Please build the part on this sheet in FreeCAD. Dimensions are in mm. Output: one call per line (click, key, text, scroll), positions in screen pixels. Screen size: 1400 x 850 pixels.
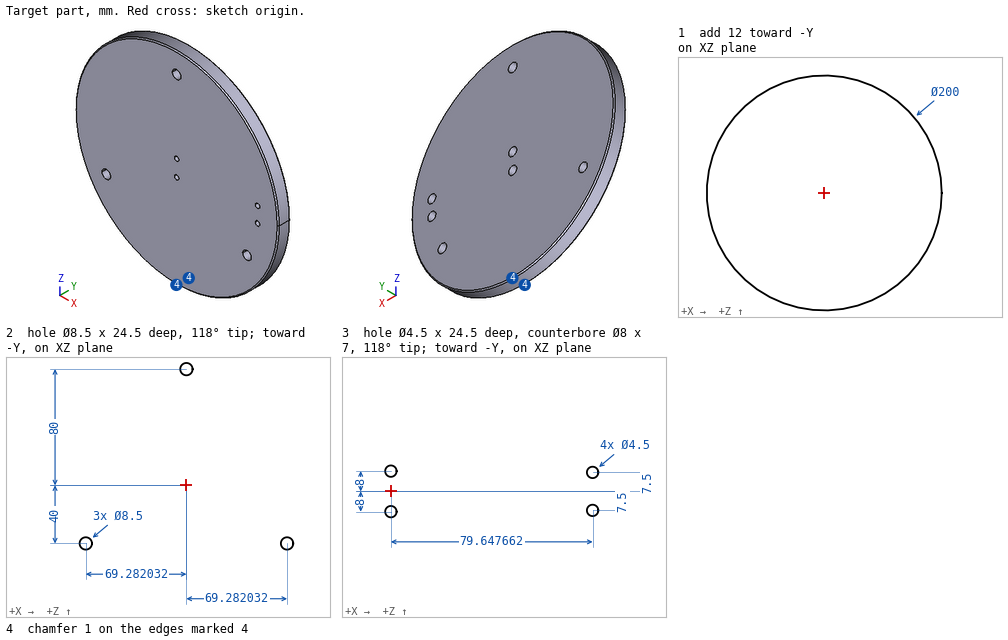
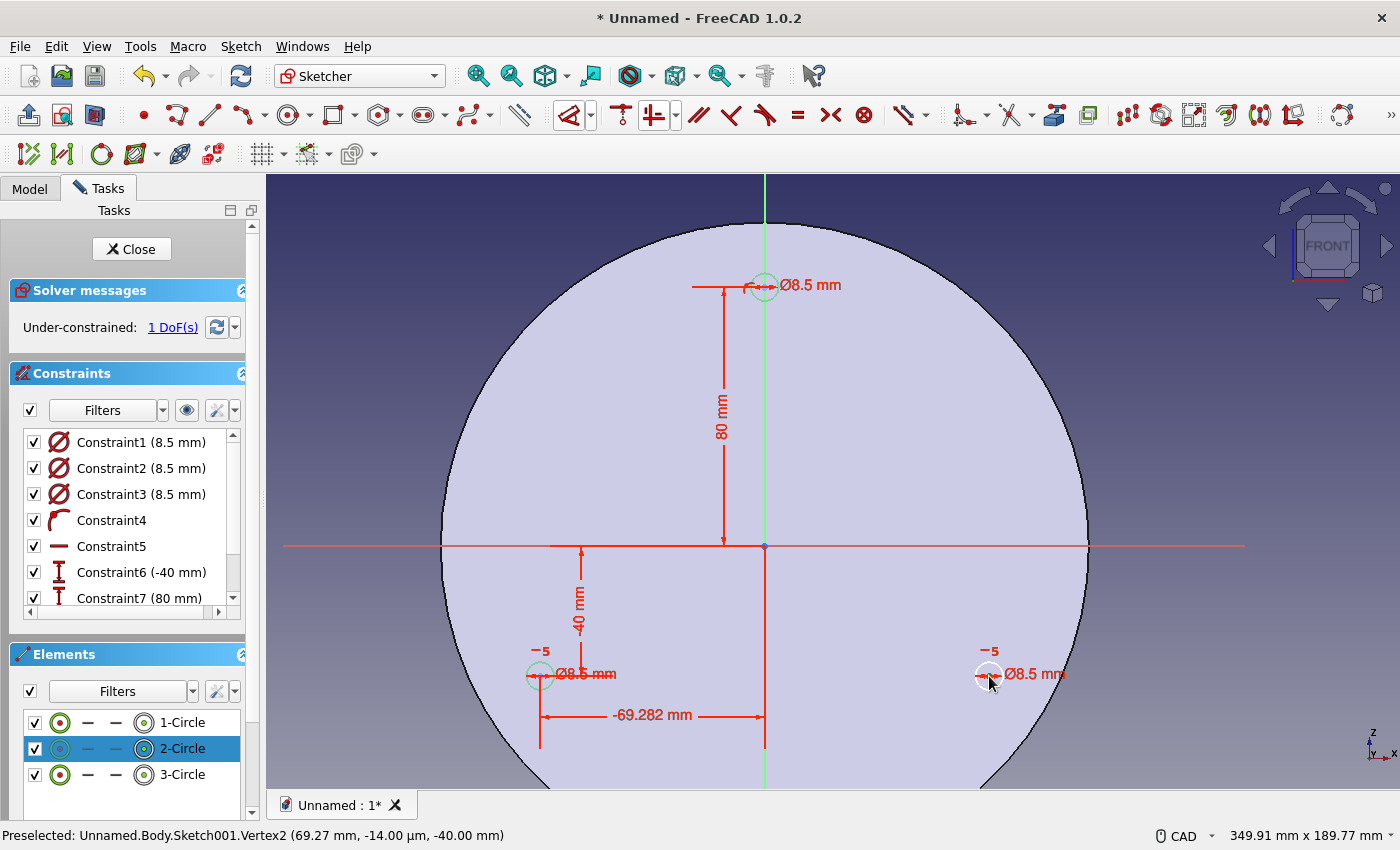
click(590, 116)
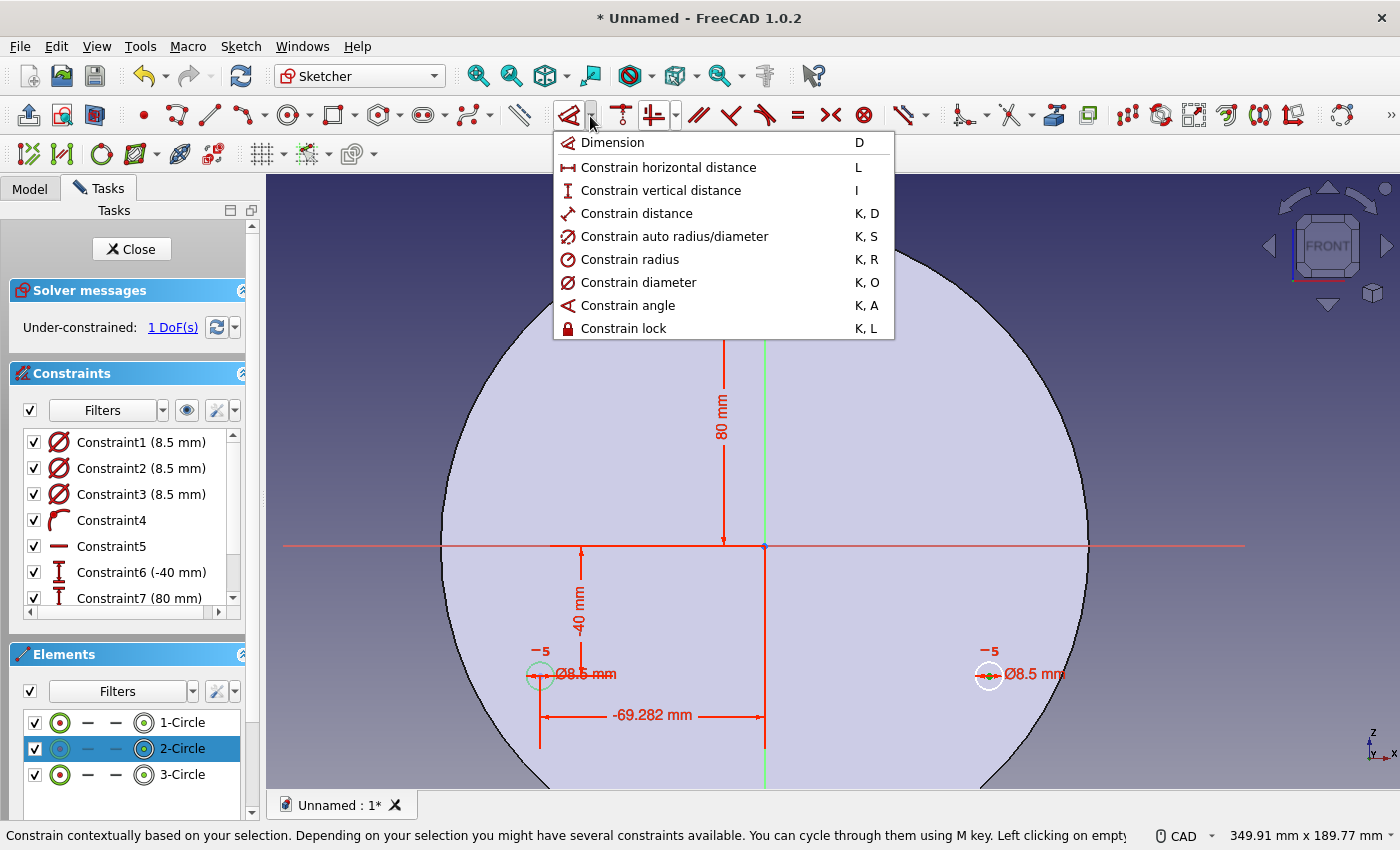
click(724, 168)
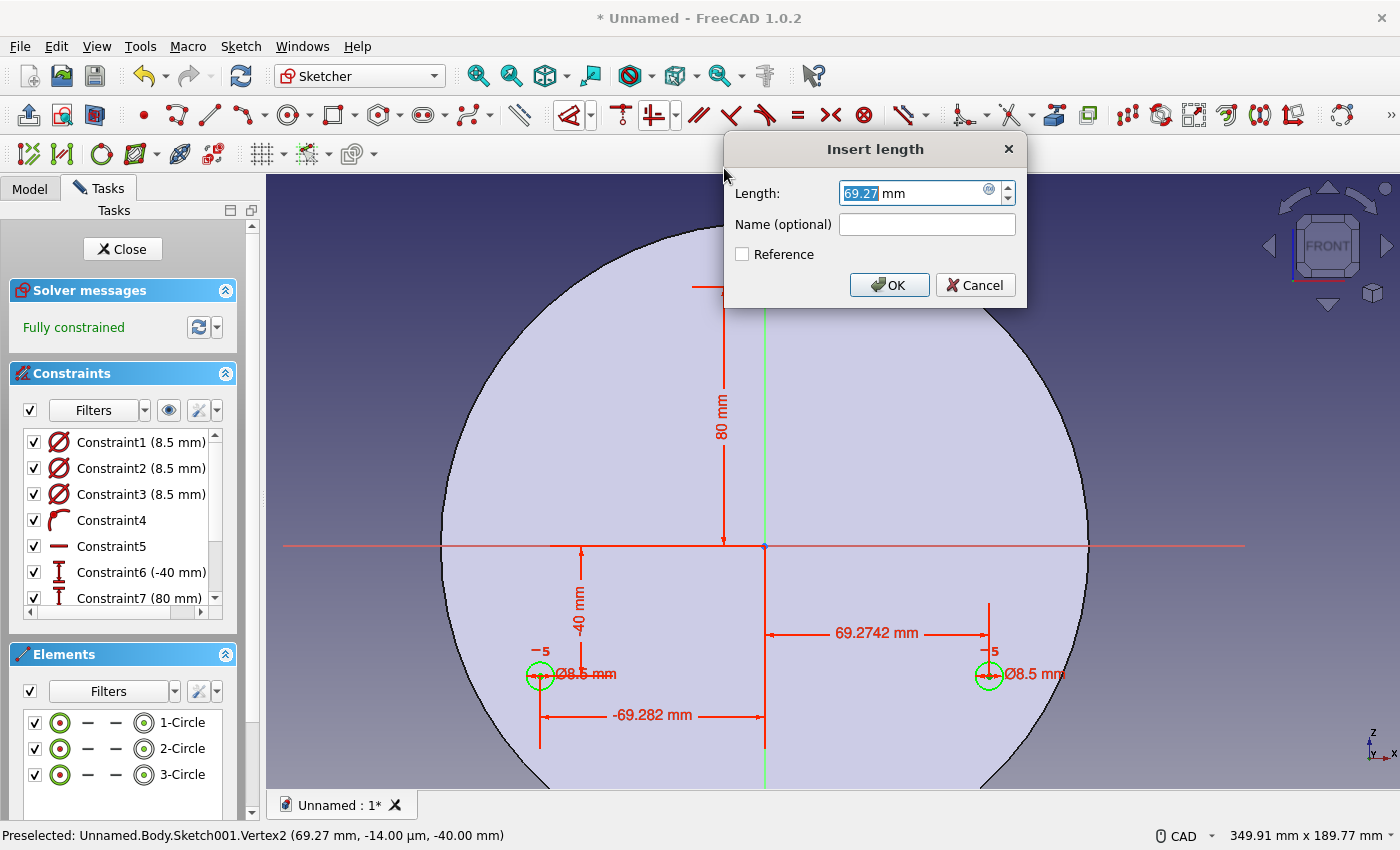
text(69.282032)
key(Return)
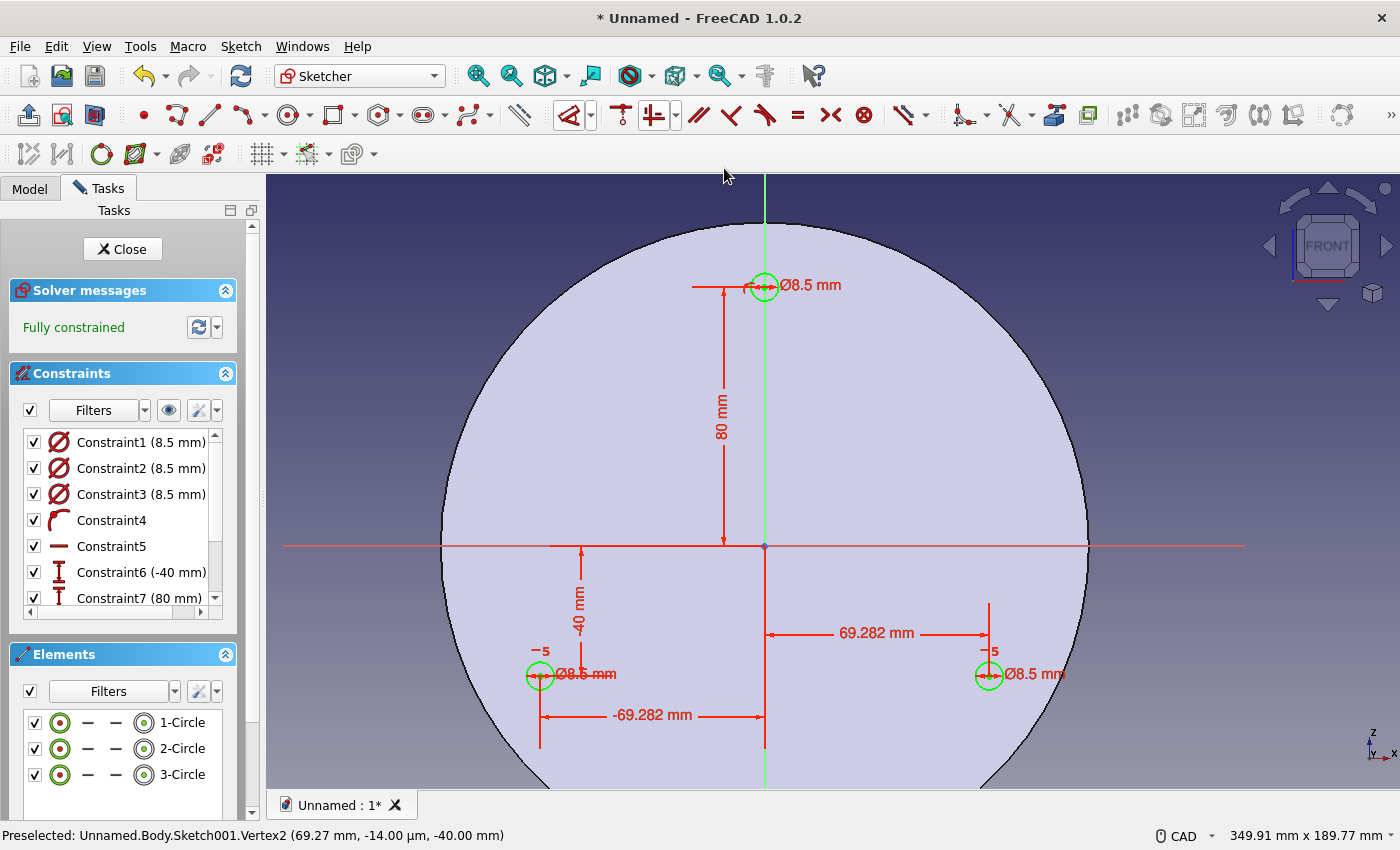
click(123, 249)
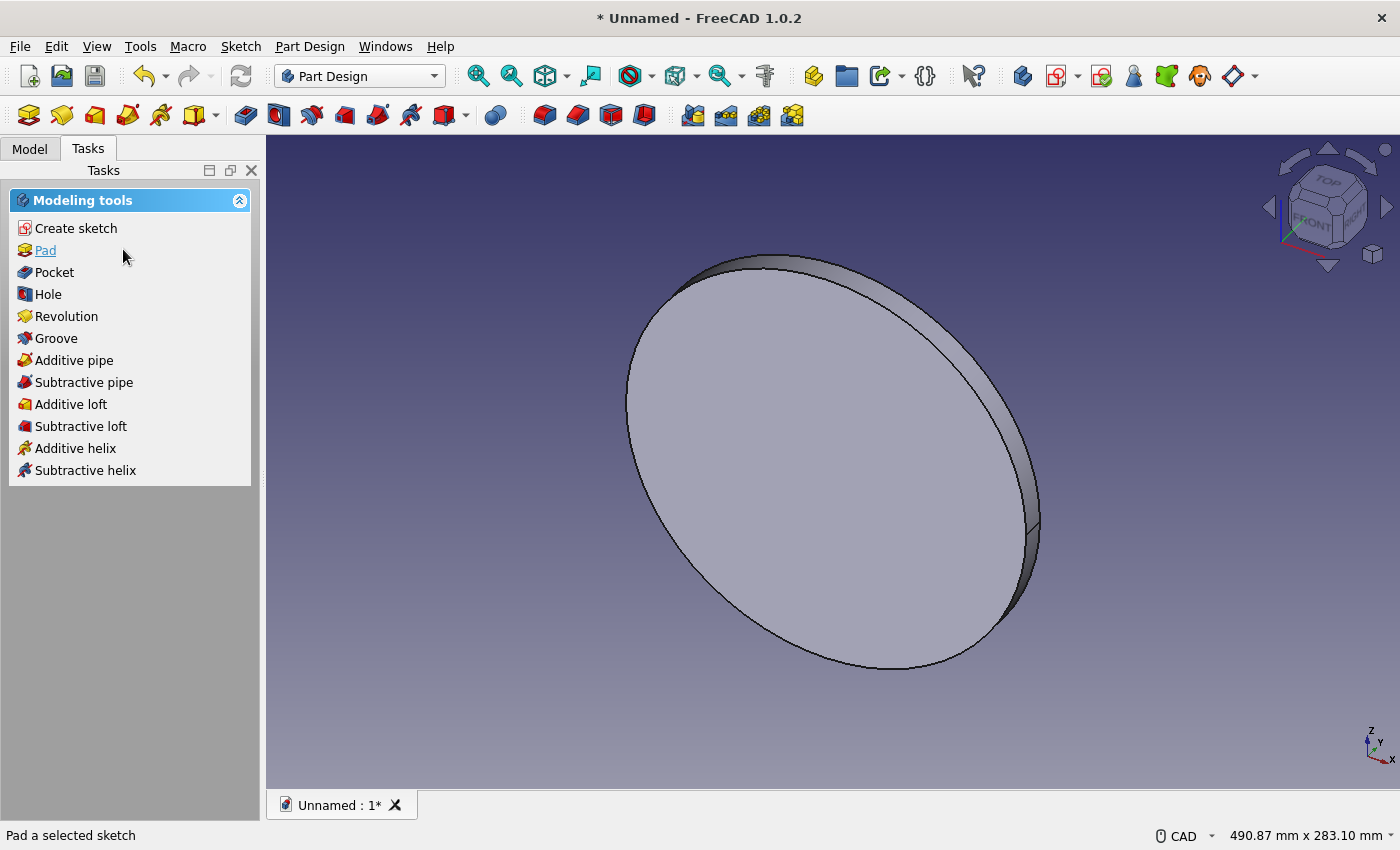
click(279, 116)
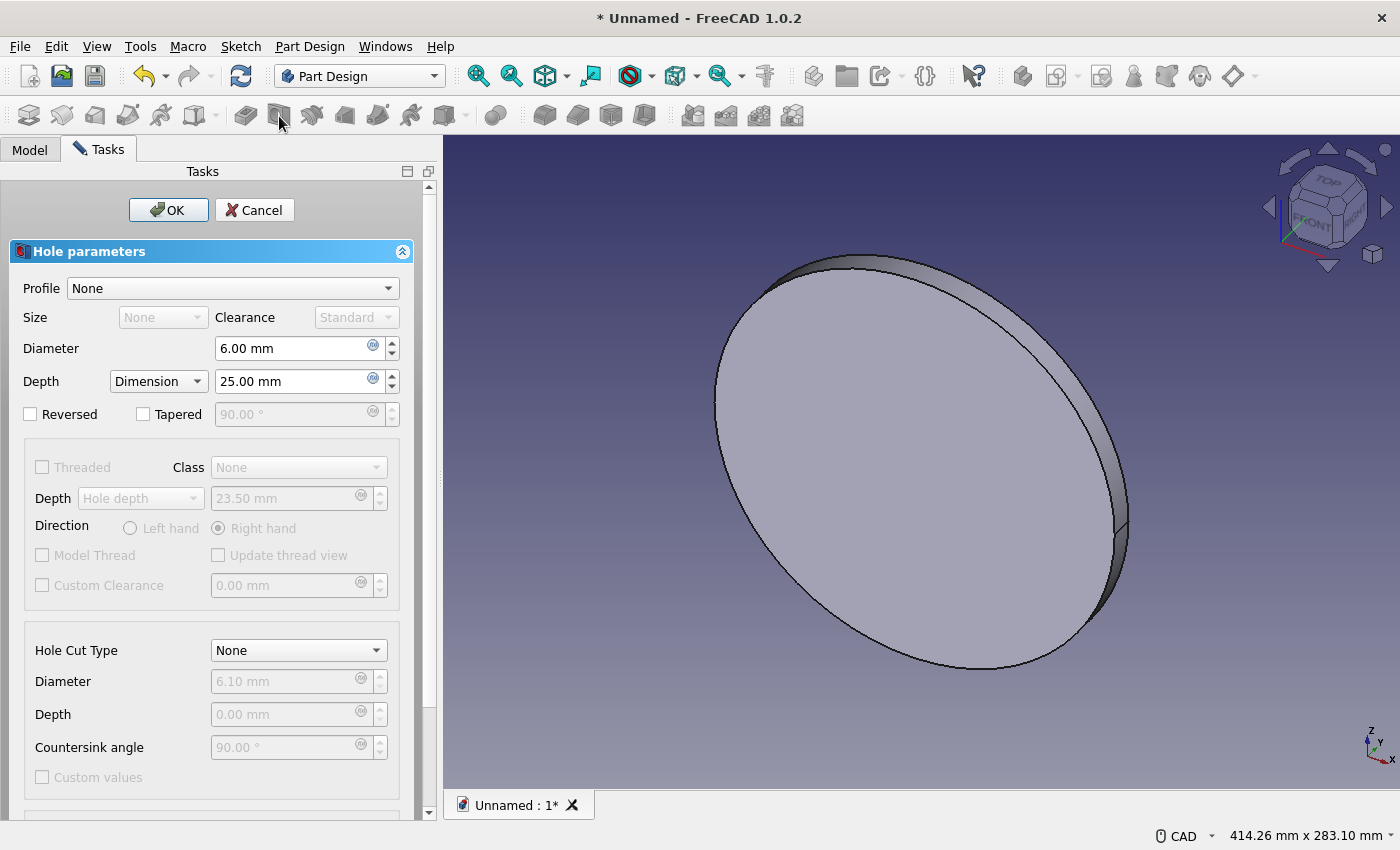
triple_click(300, 348)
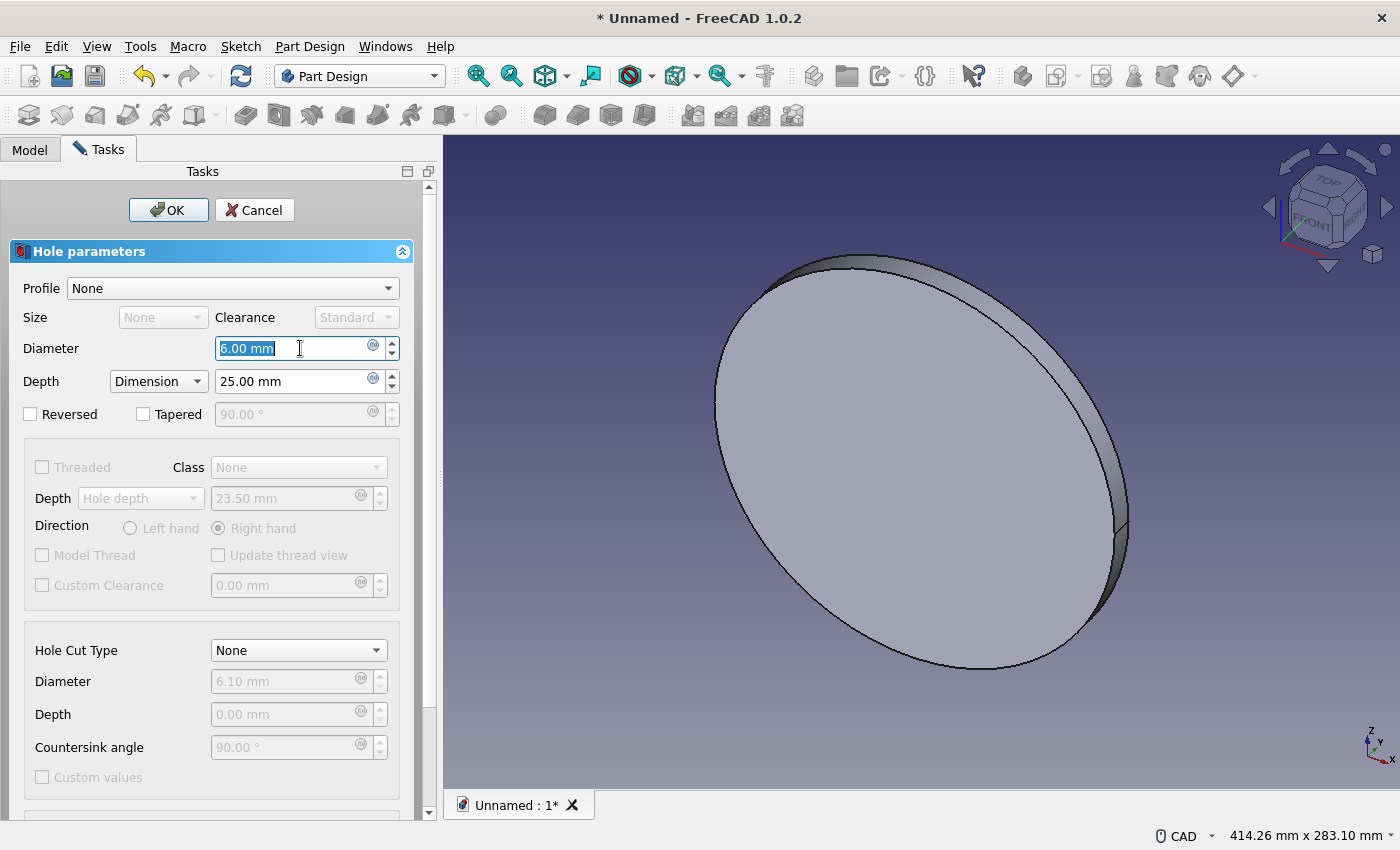
text(8.5)
key(Tab)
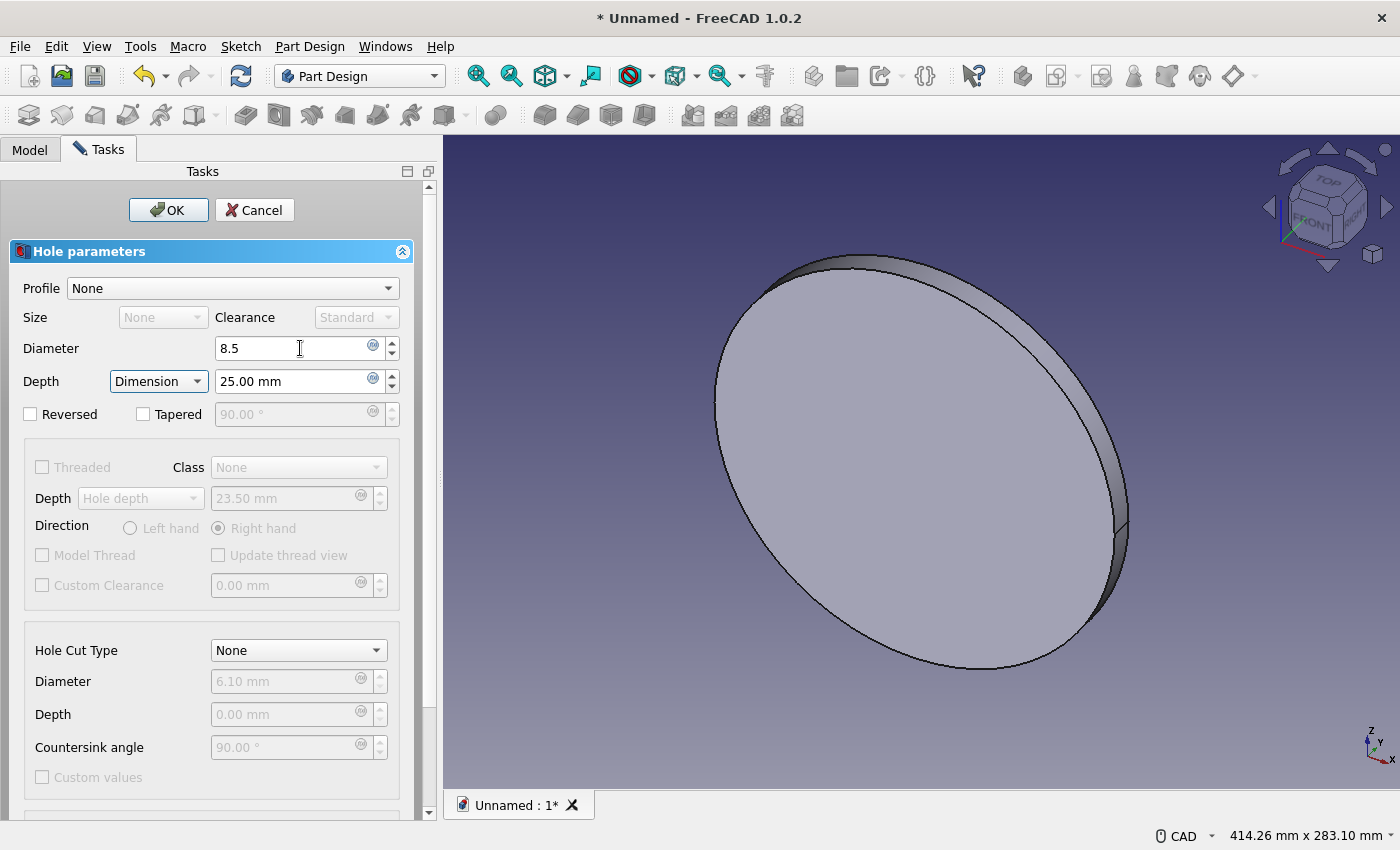
triple_click(300, 382)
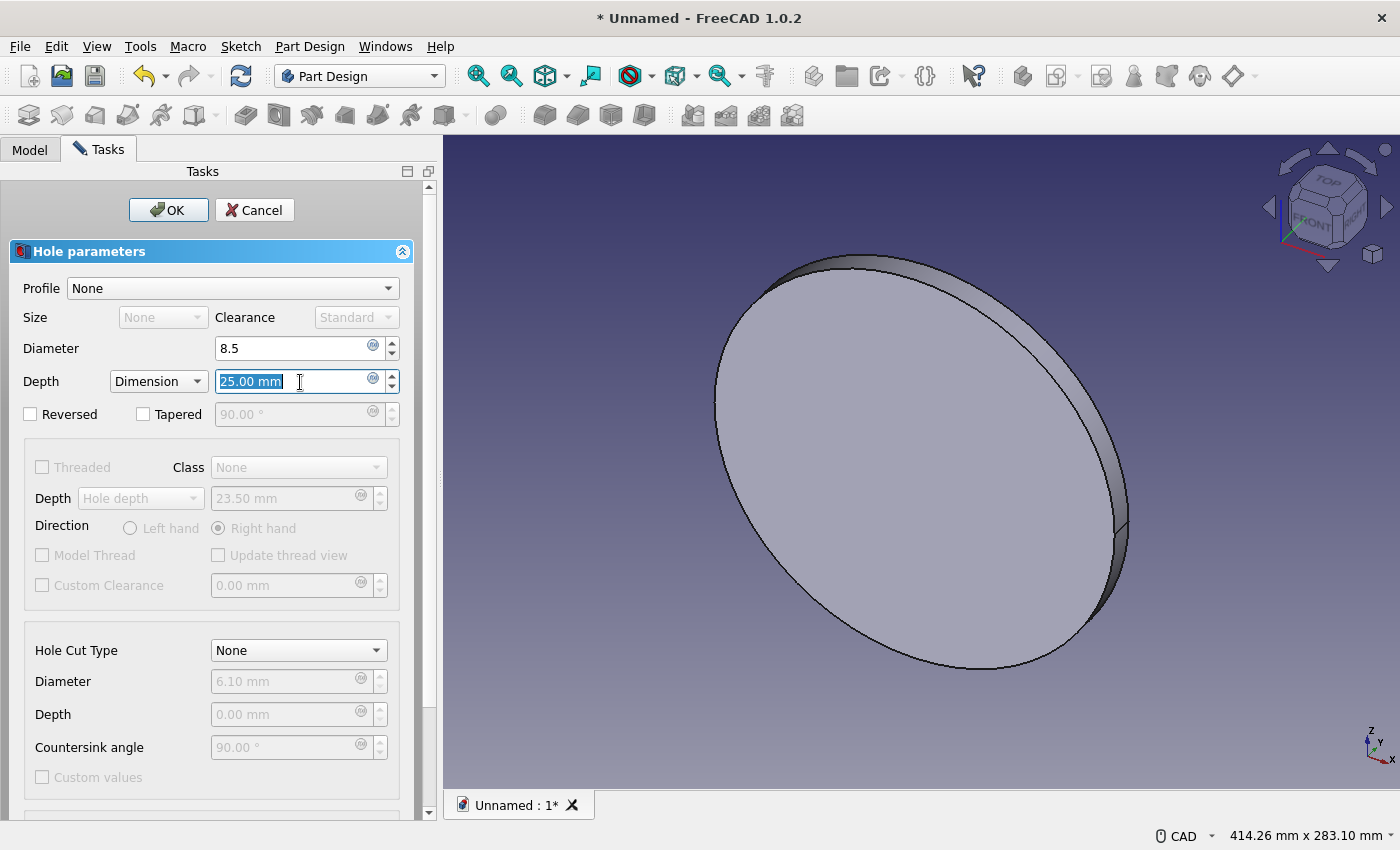
text(24.5)
key(Tab)